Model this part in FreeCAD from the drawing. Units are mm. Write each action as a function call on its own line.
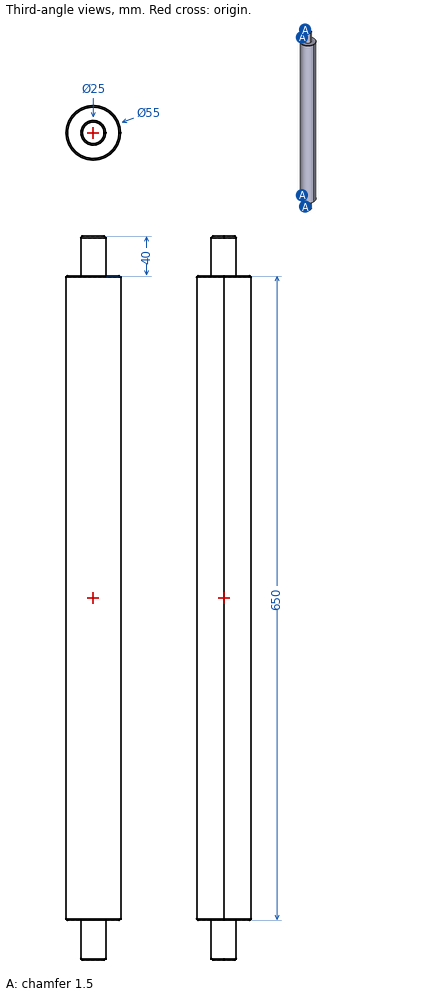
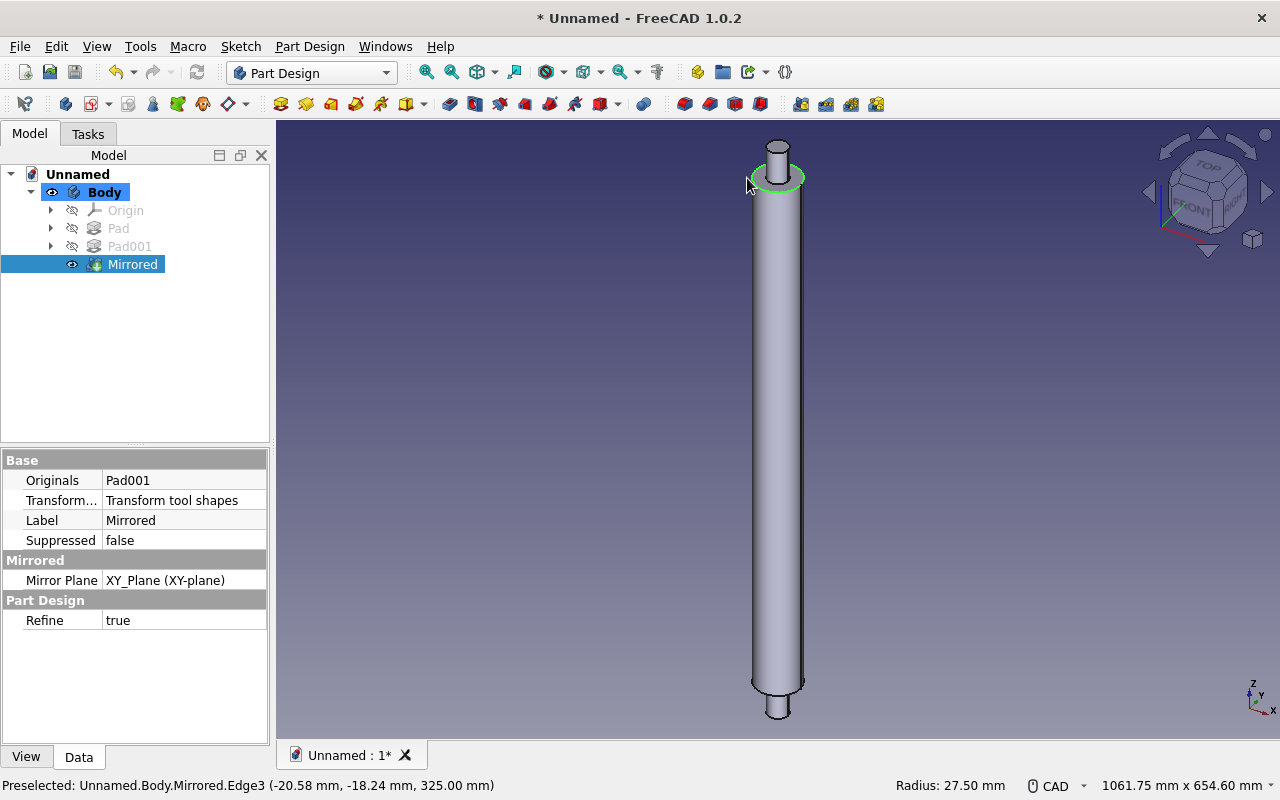
click(769, 150, ctrl)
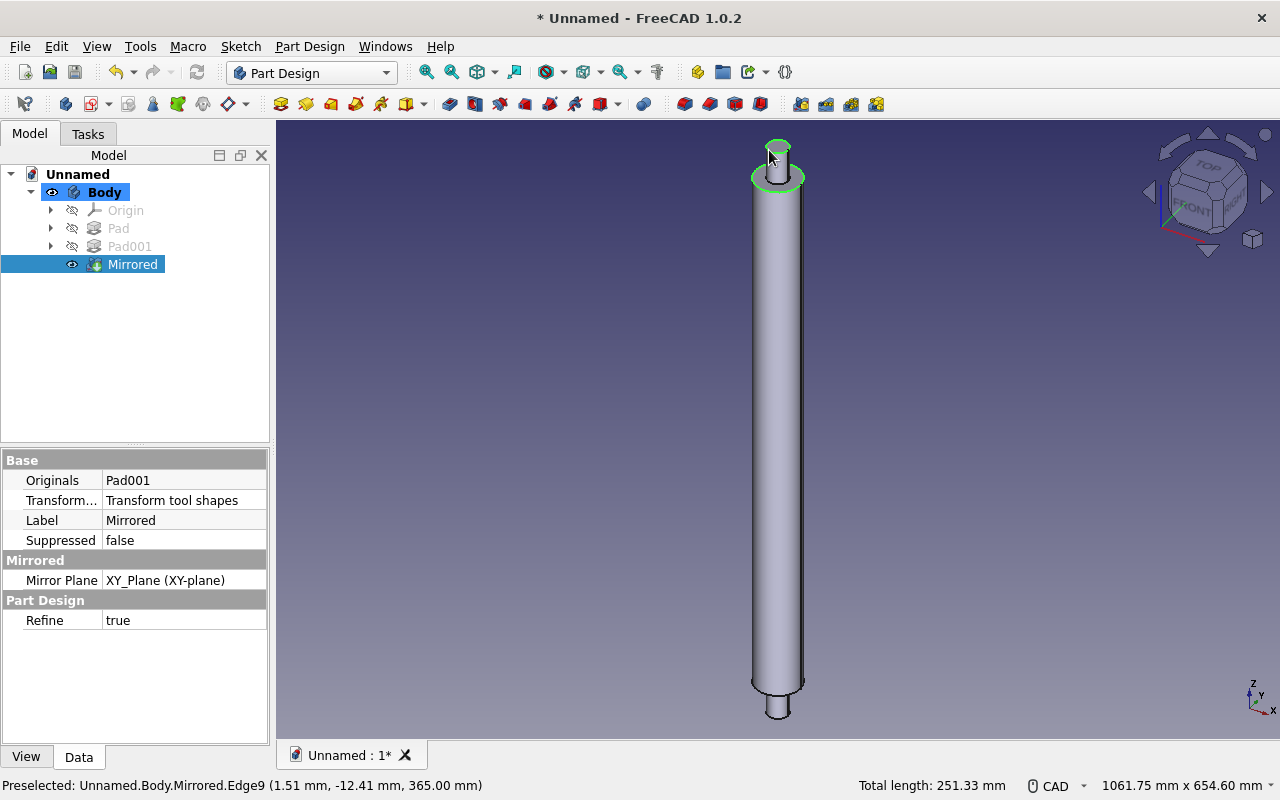
key(0)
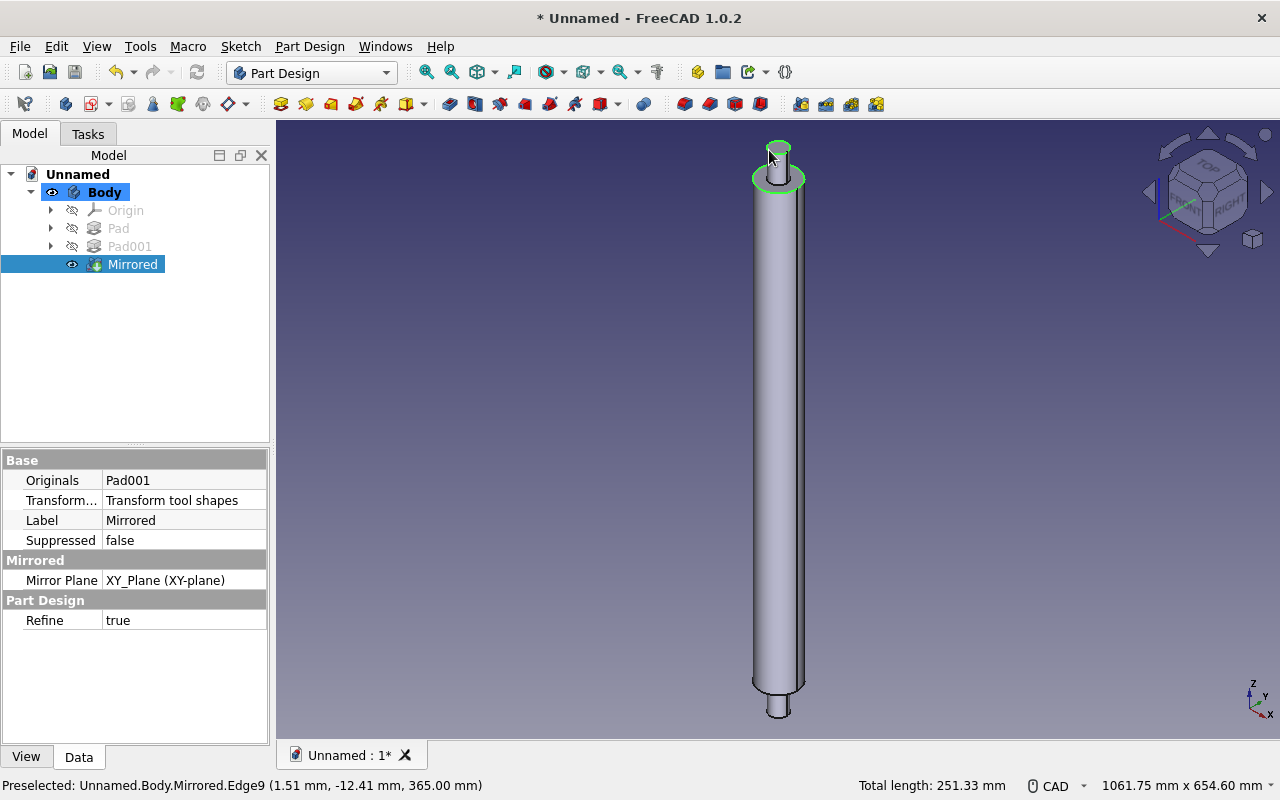
click(755, 686, ctrl)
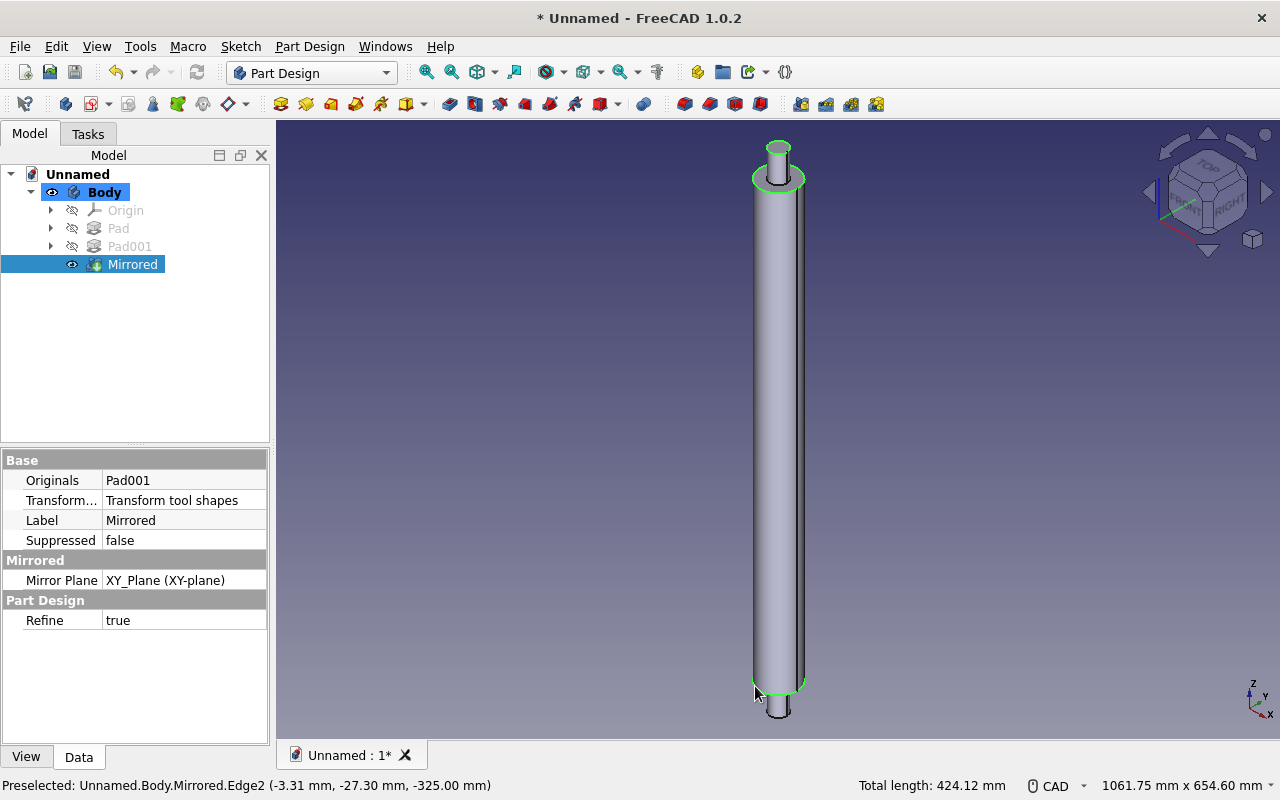
key(2)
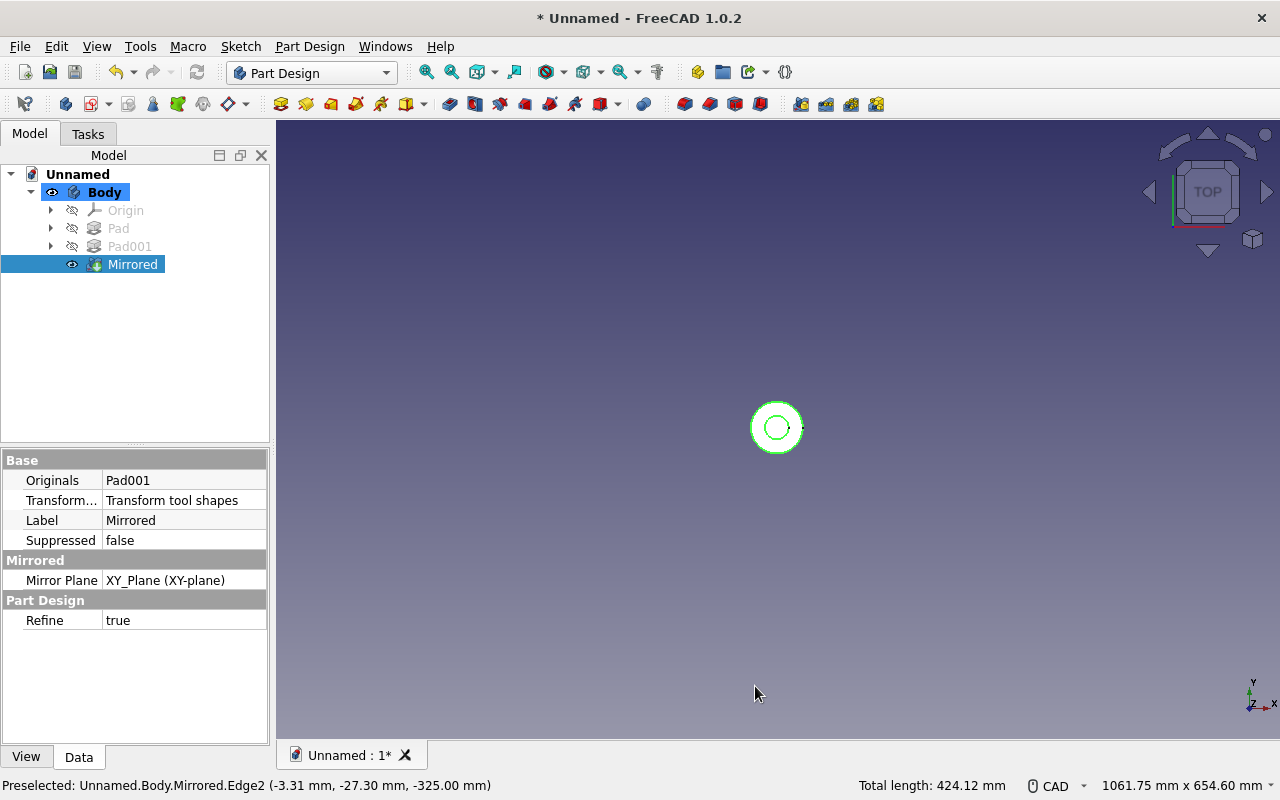
key(v)
key(f)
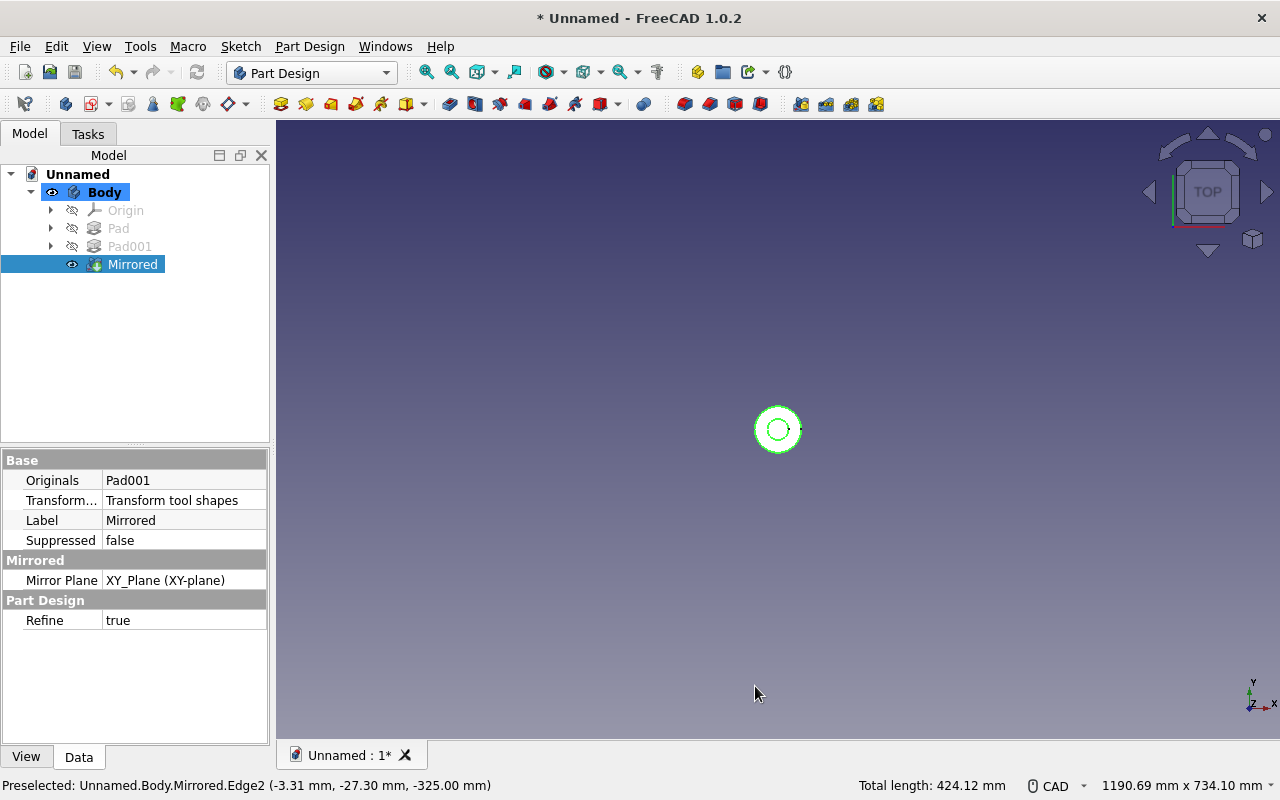
key(1)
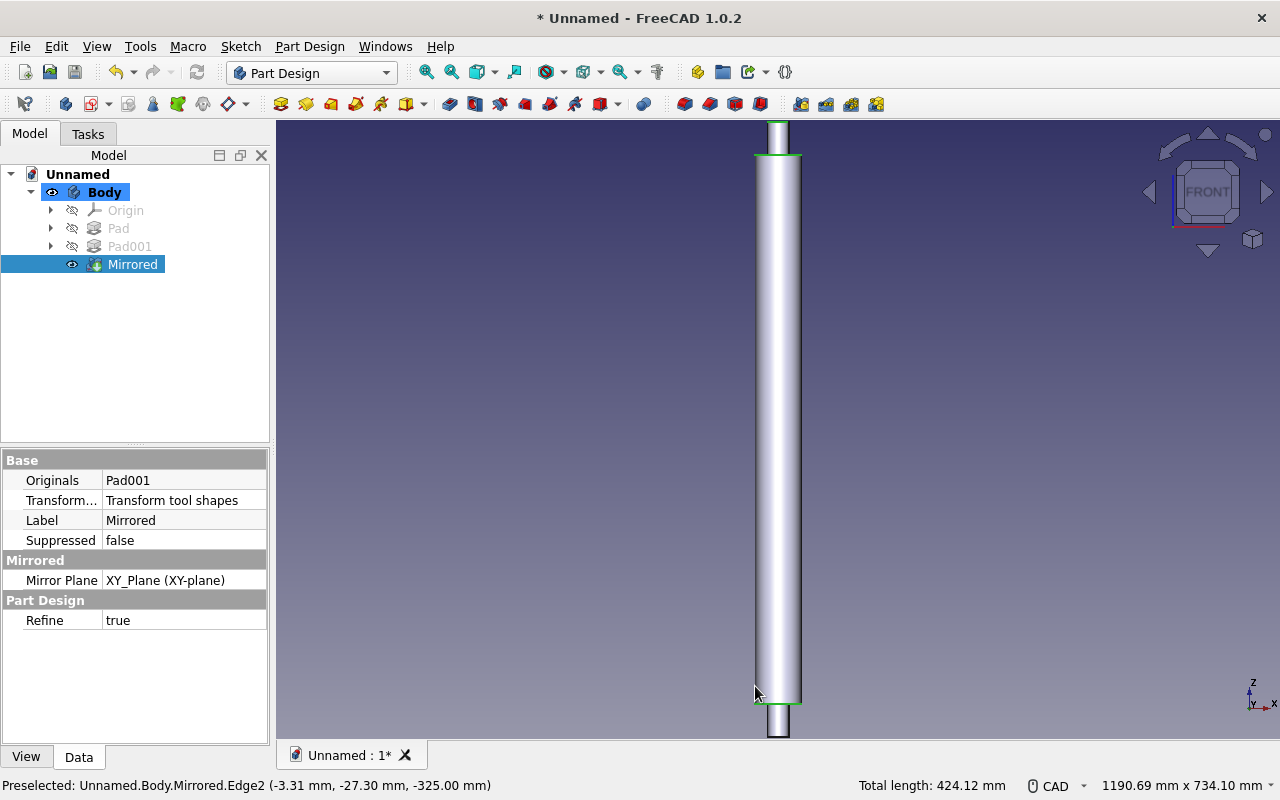
key(3)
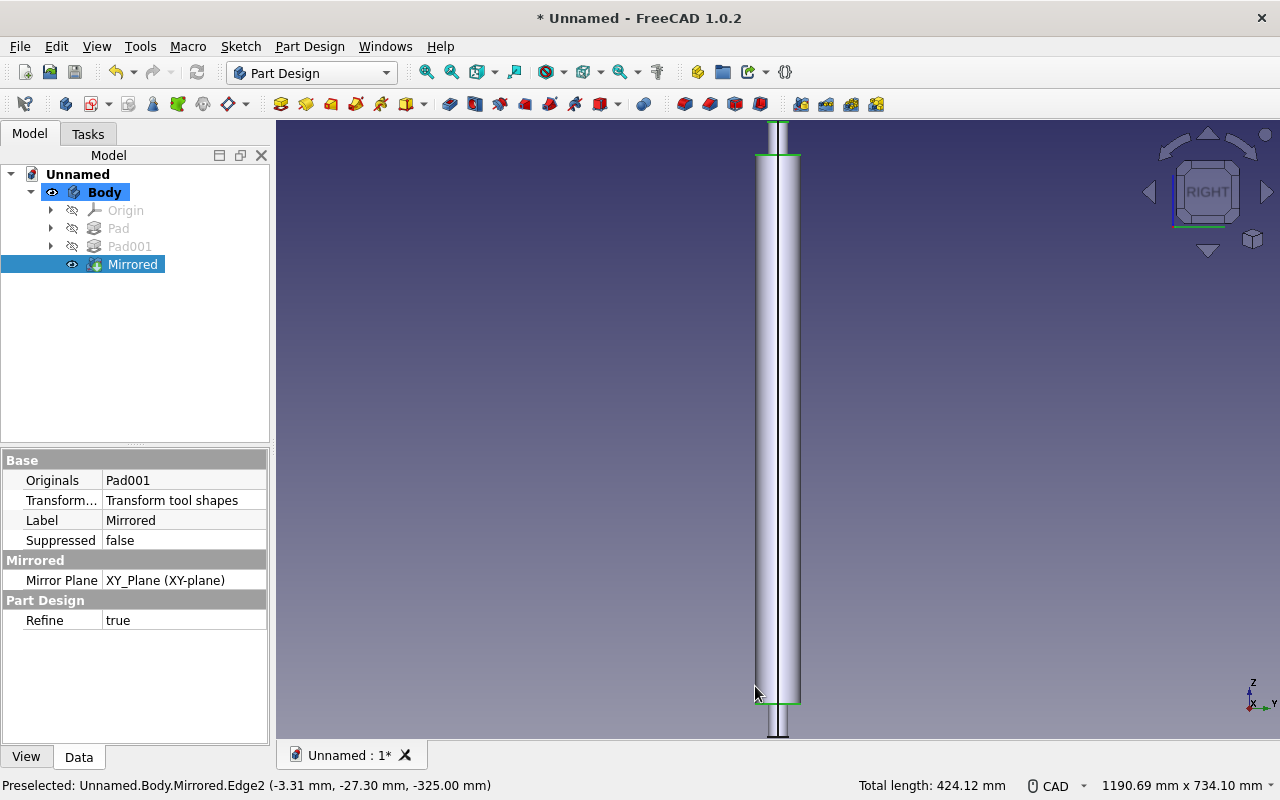
key(5)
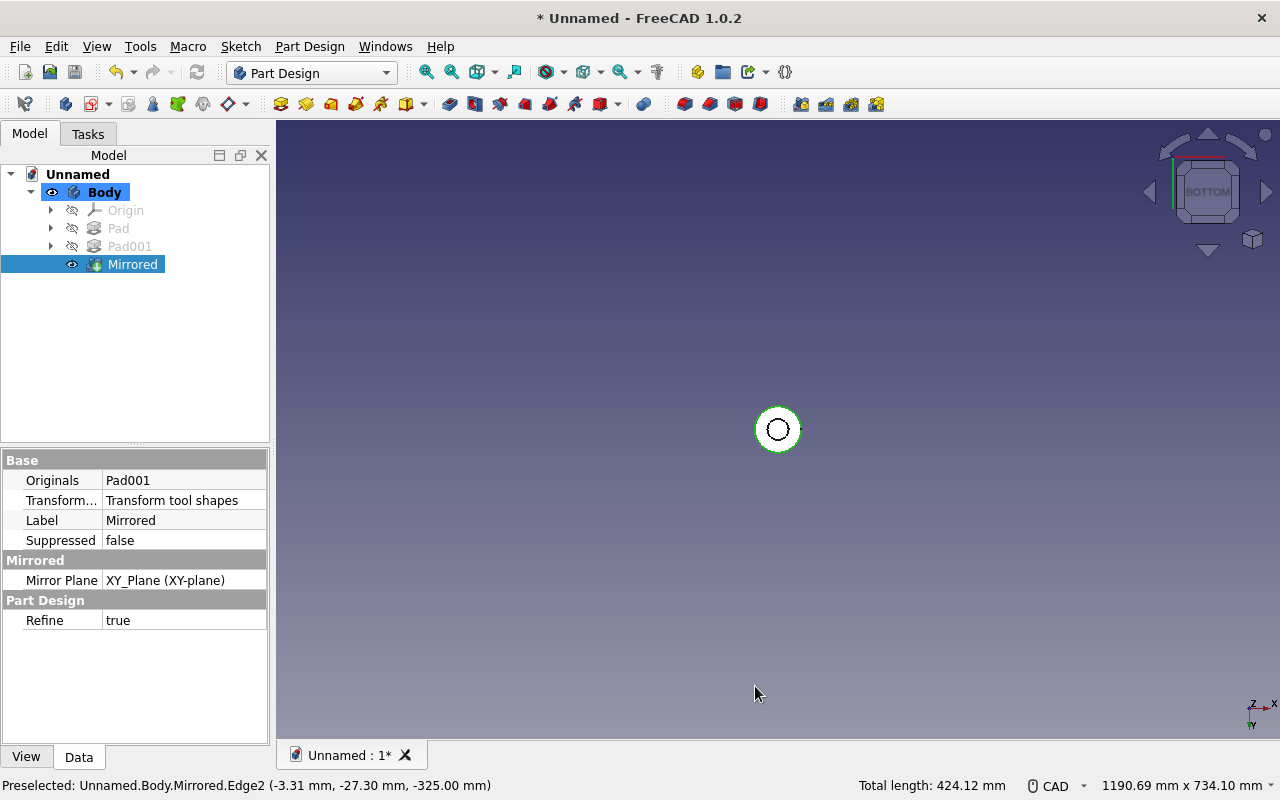
key(v)
key(f)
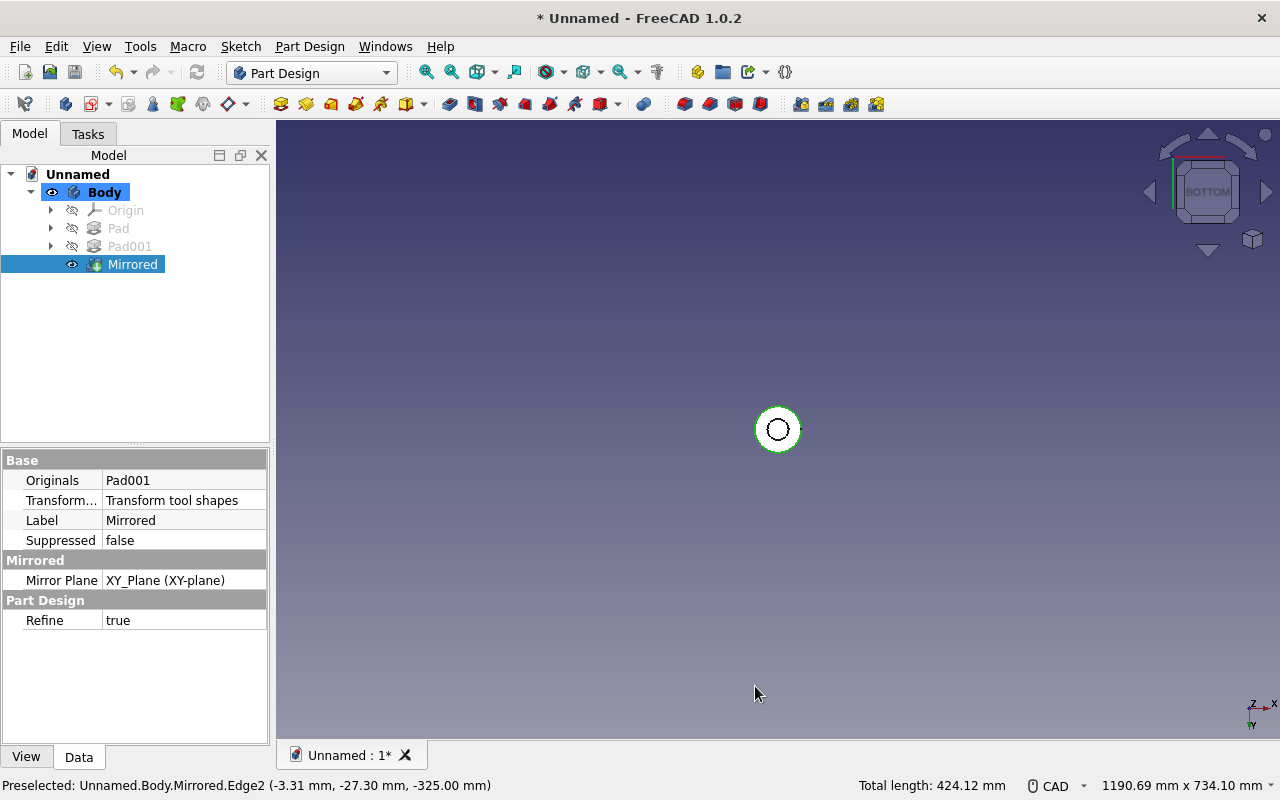
click(767, 428, ctrl)